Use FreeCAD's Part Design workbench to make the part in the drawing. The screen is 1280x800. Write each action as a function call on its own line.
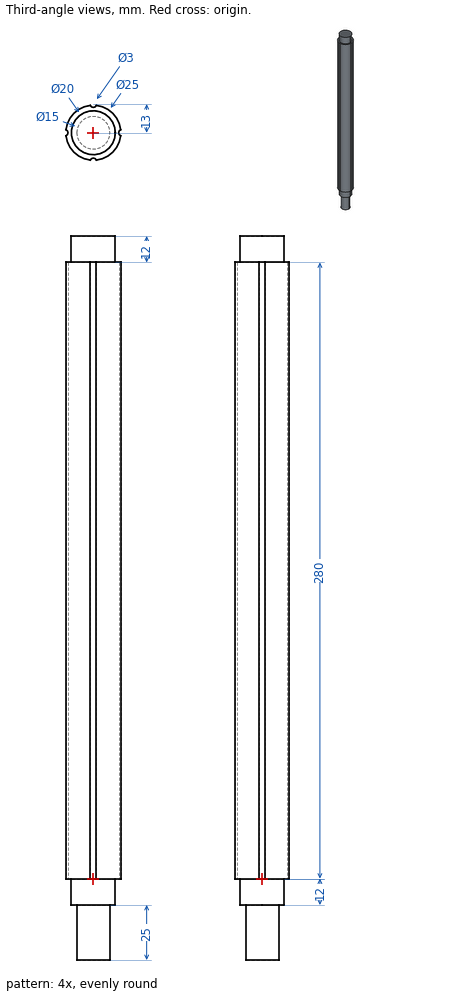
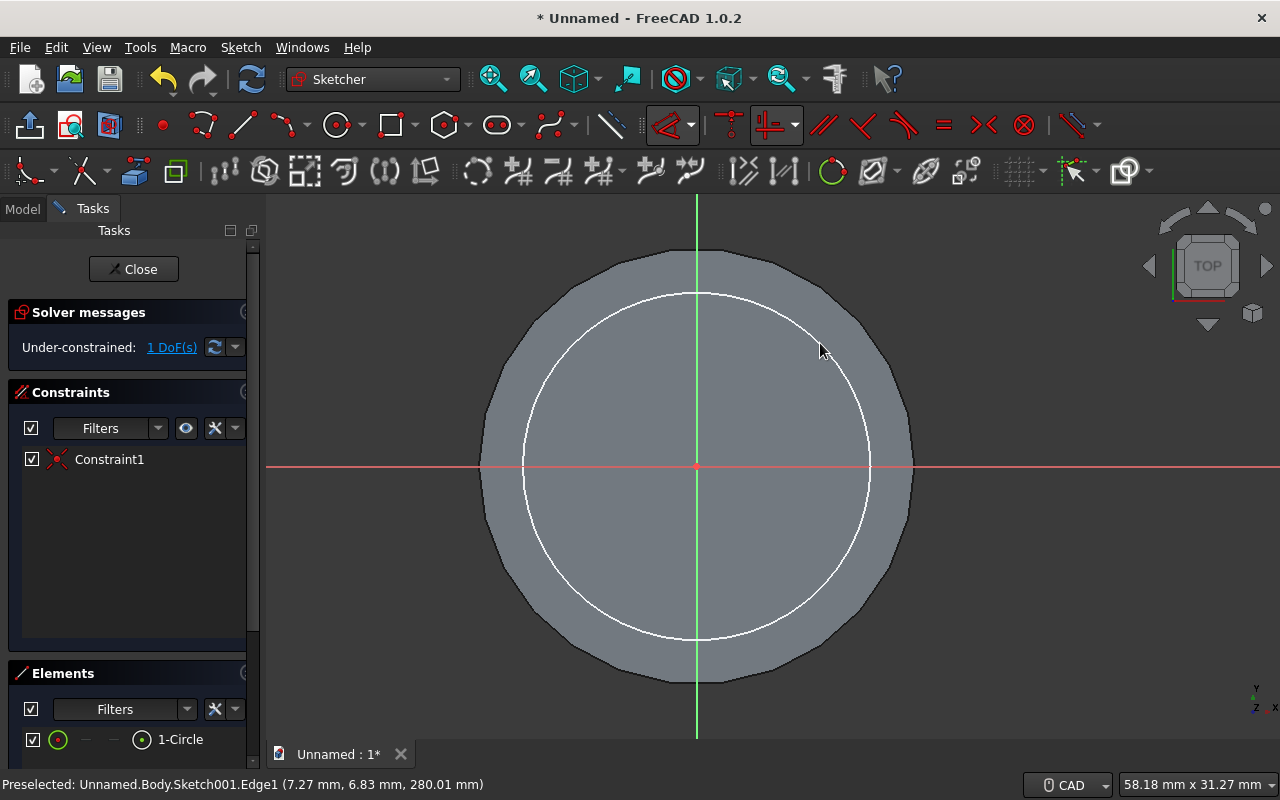
click(666, 126)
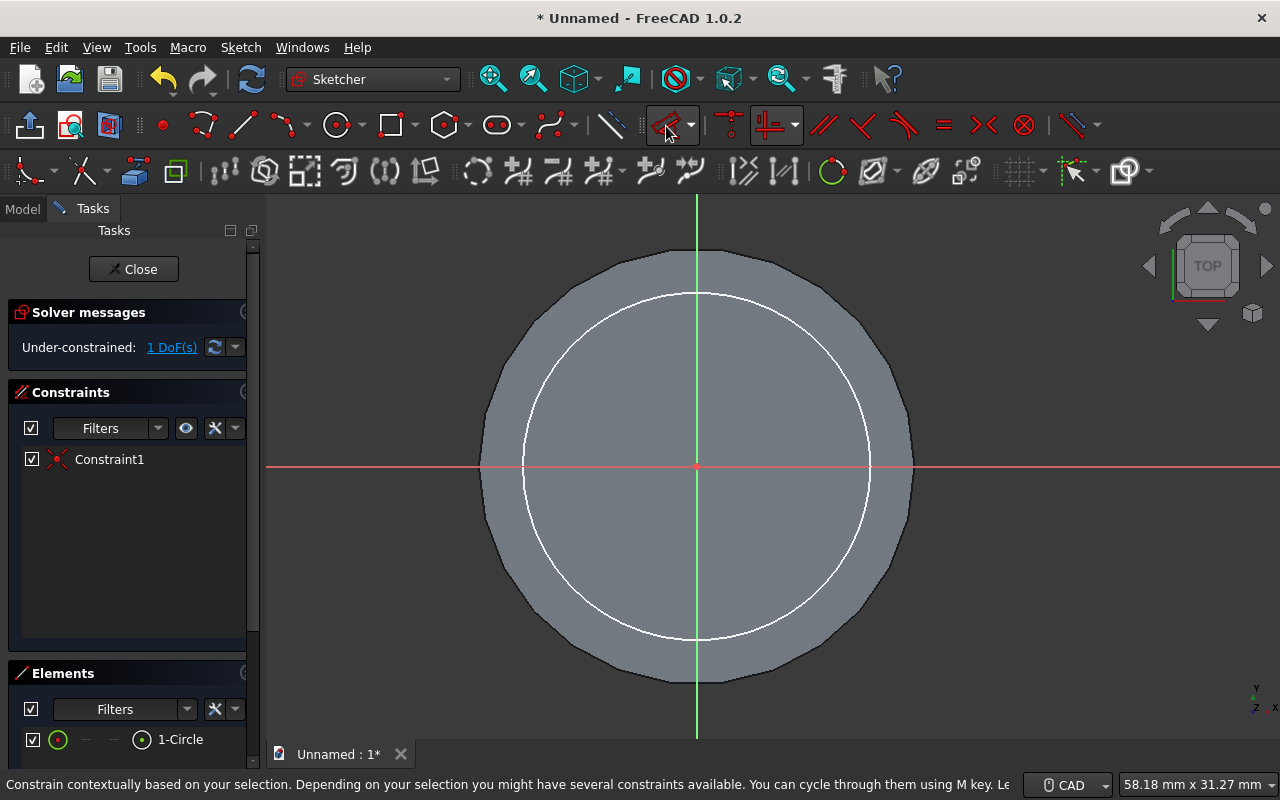
click(819, 343)
click(842, 320)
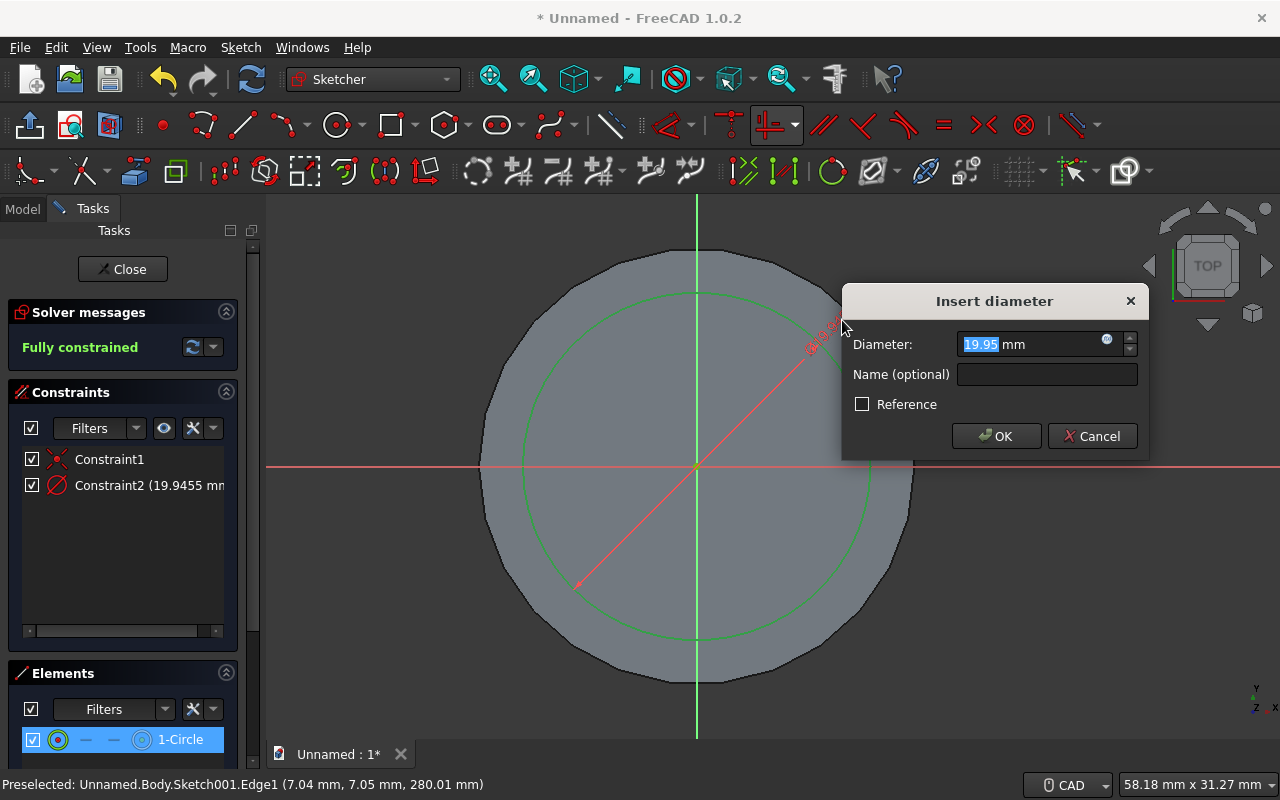
text(20)
key(Return)
key(Escape)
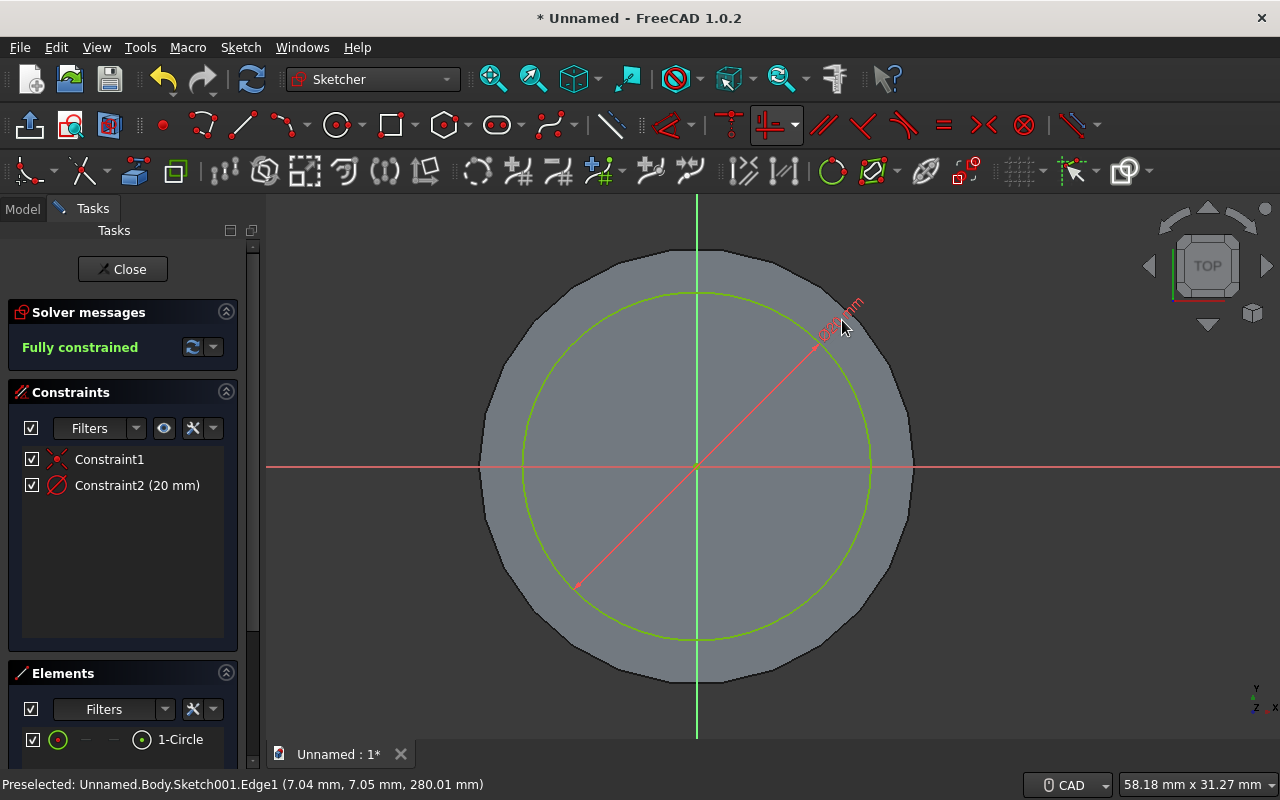
click(123, 269)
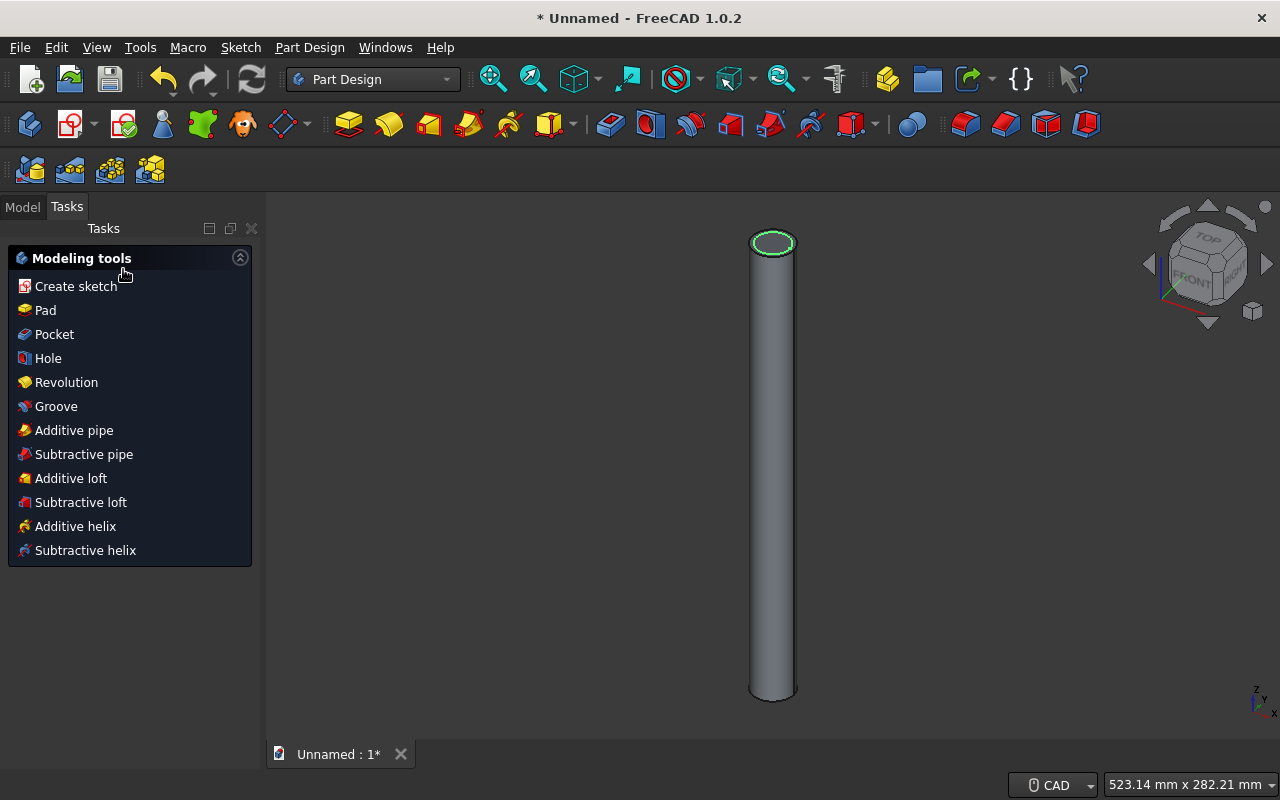
click(350, 124)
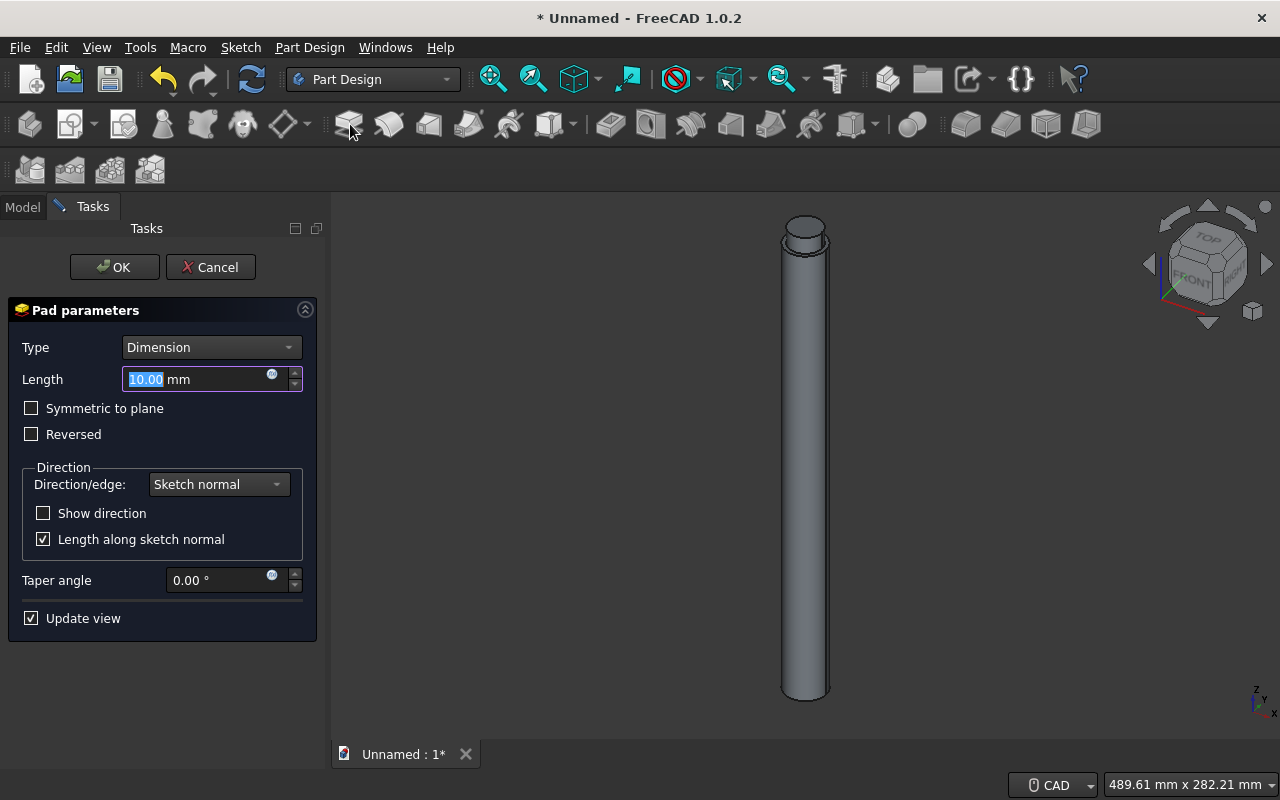
text(12)
key(Tab)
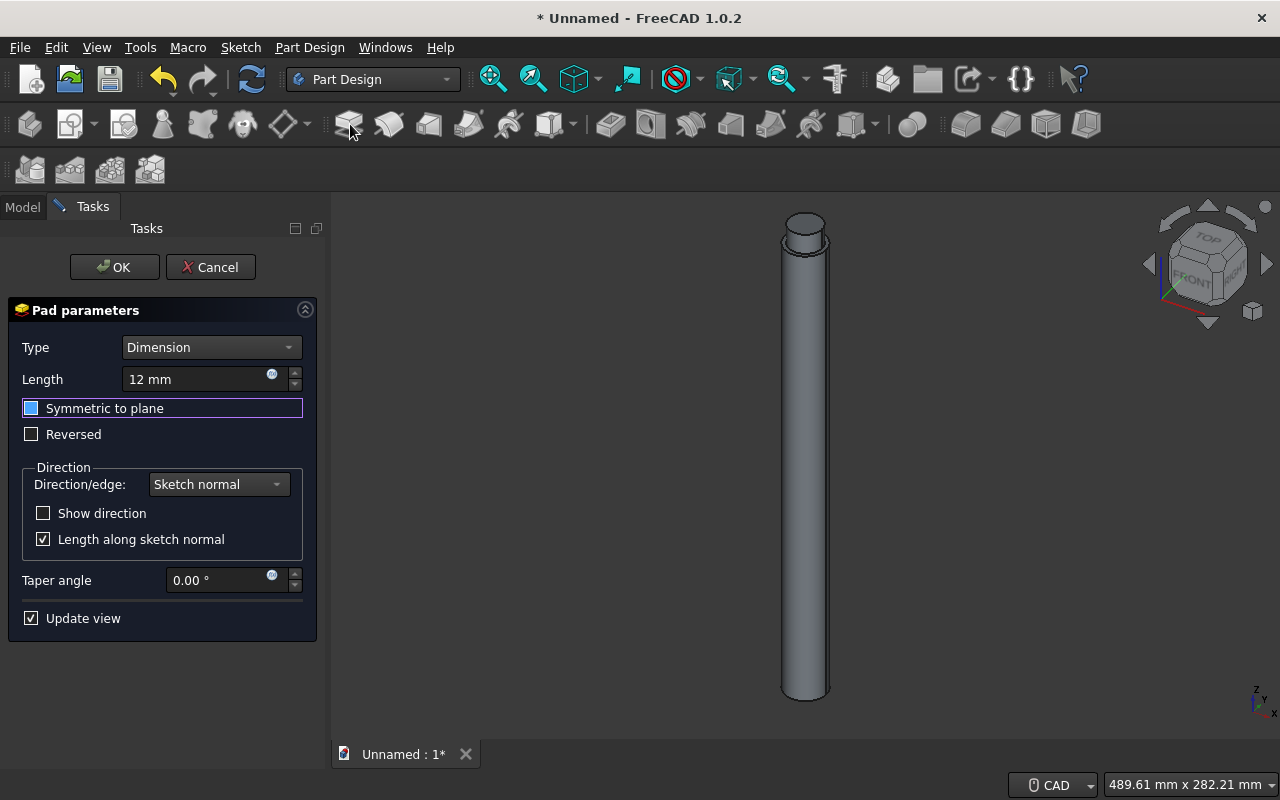
click(115, 267)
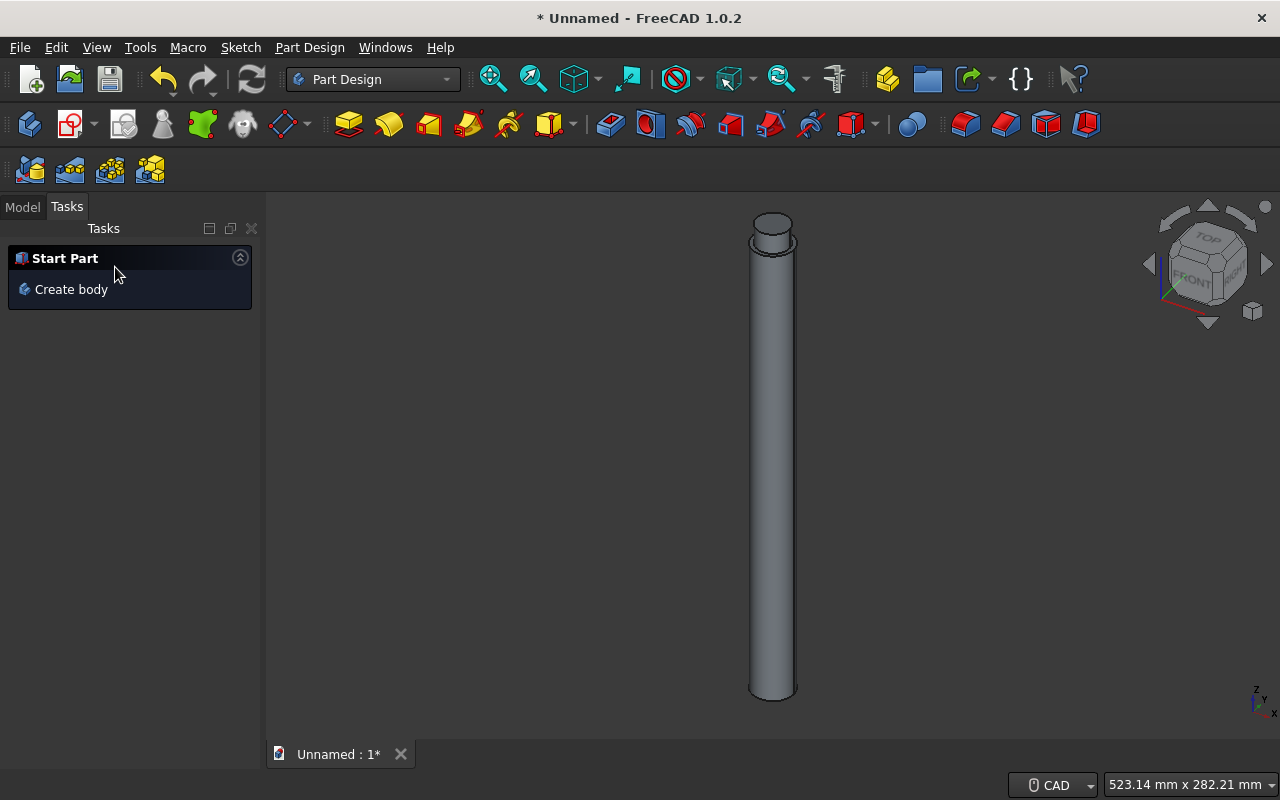
click(23, 206)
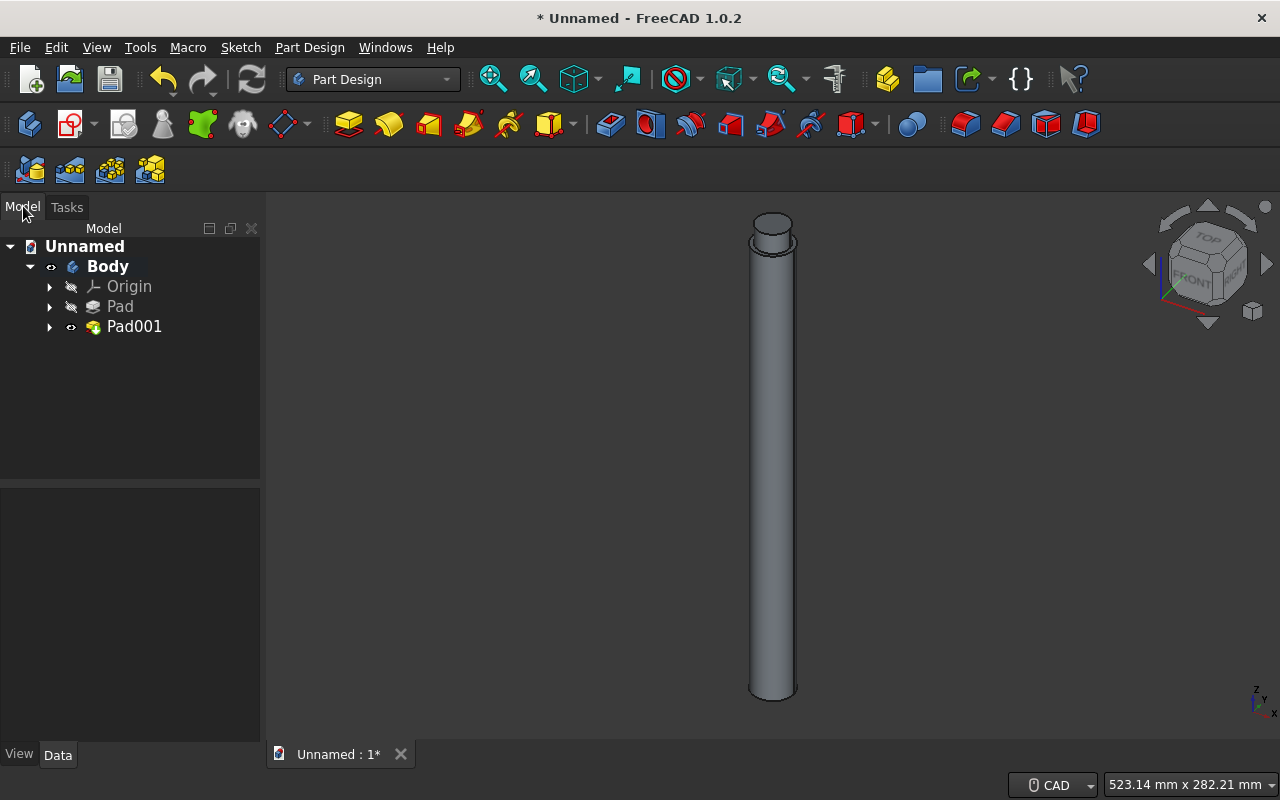
click(50, 287)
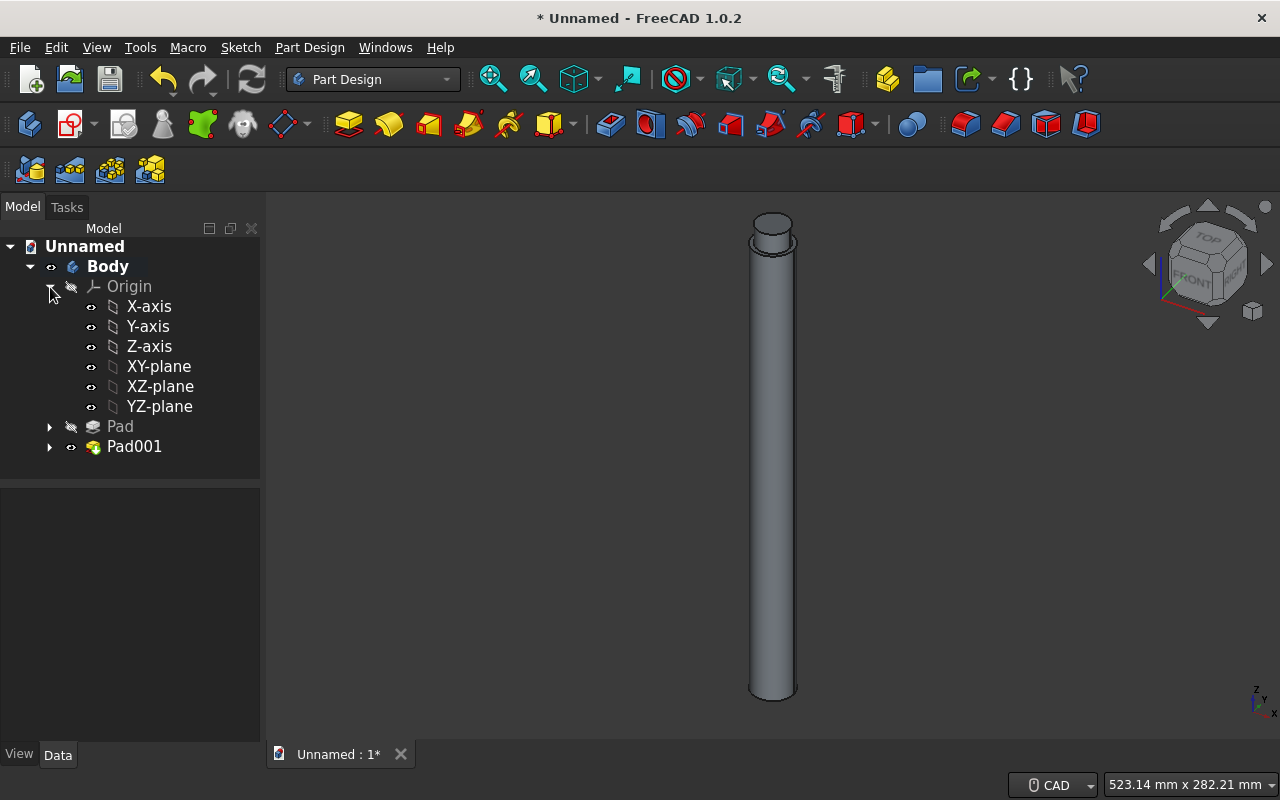
click(136, 367)